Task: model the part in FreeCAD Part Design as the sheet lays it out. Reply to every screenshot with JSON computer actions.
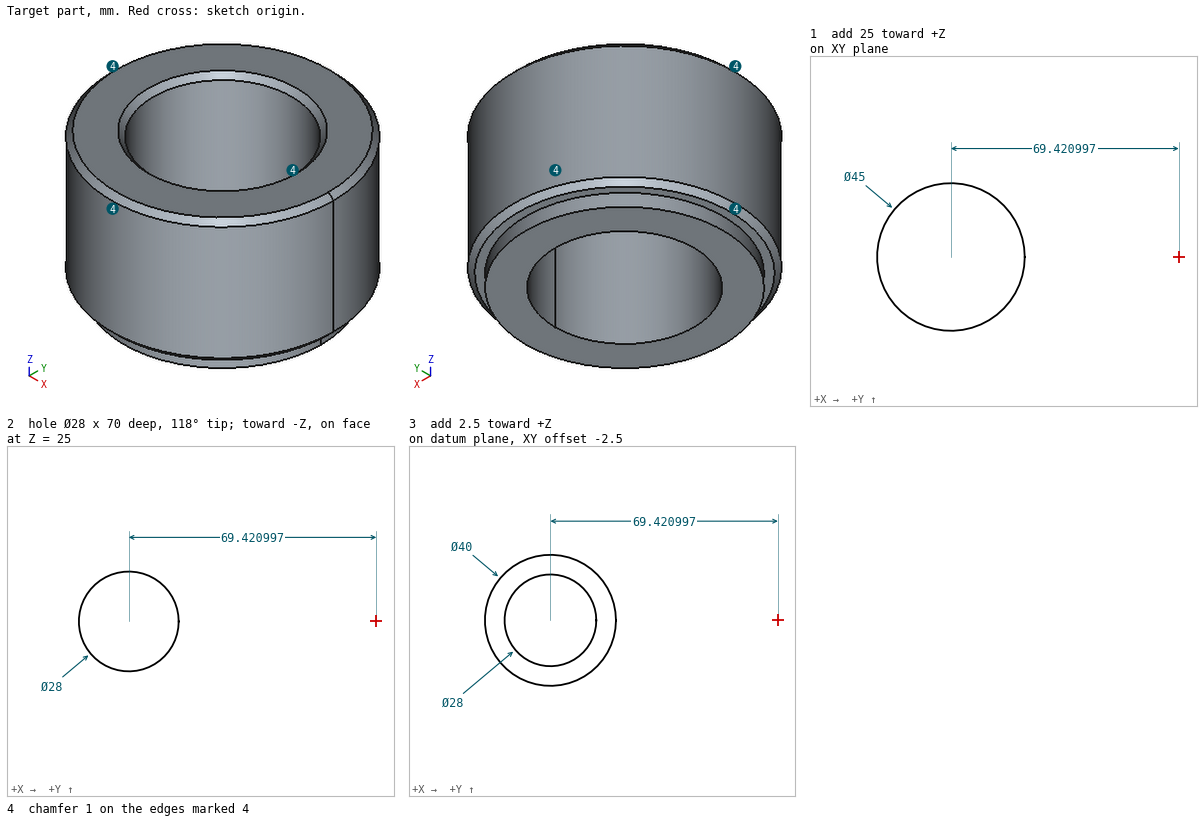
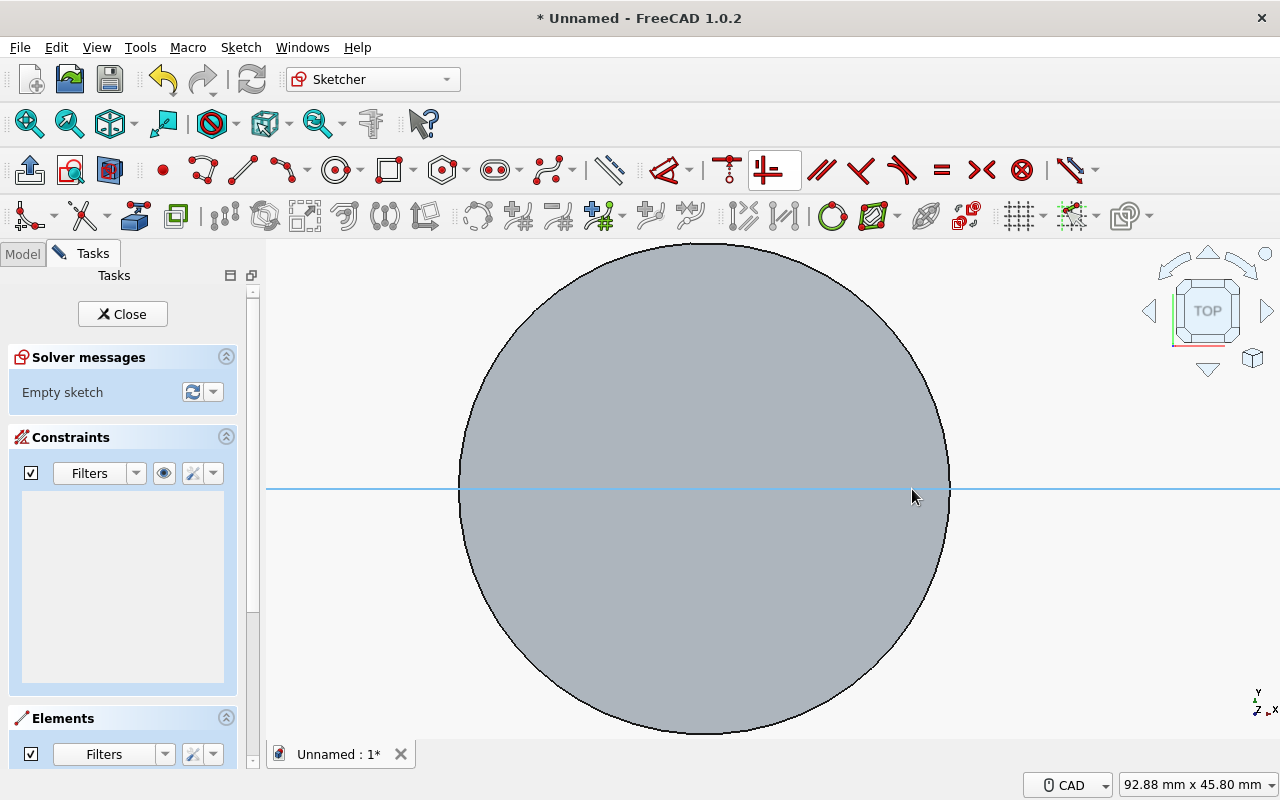
{"action": "key", "text": "g c"}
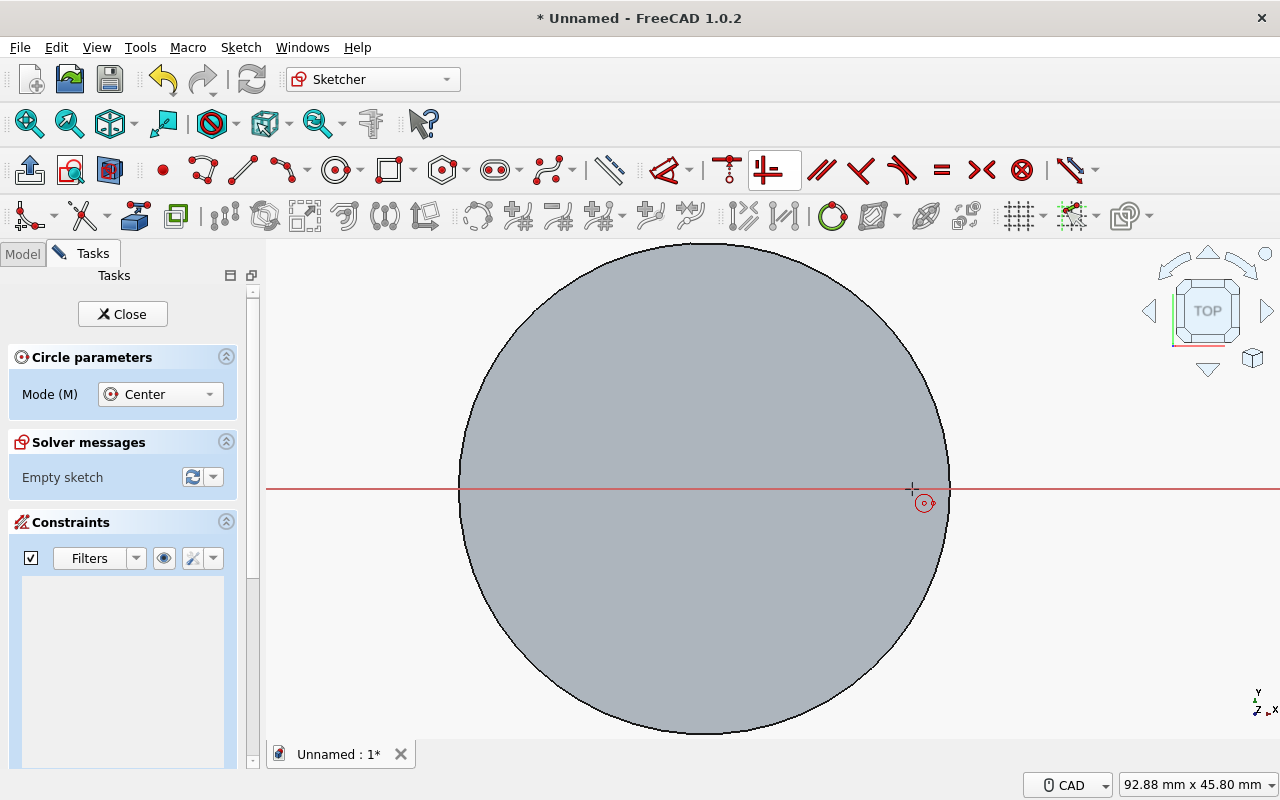
{"action": "left_click", "coordinate": [704, 489]}
{"action": "mouse_move", "coordinate": [812, 381]}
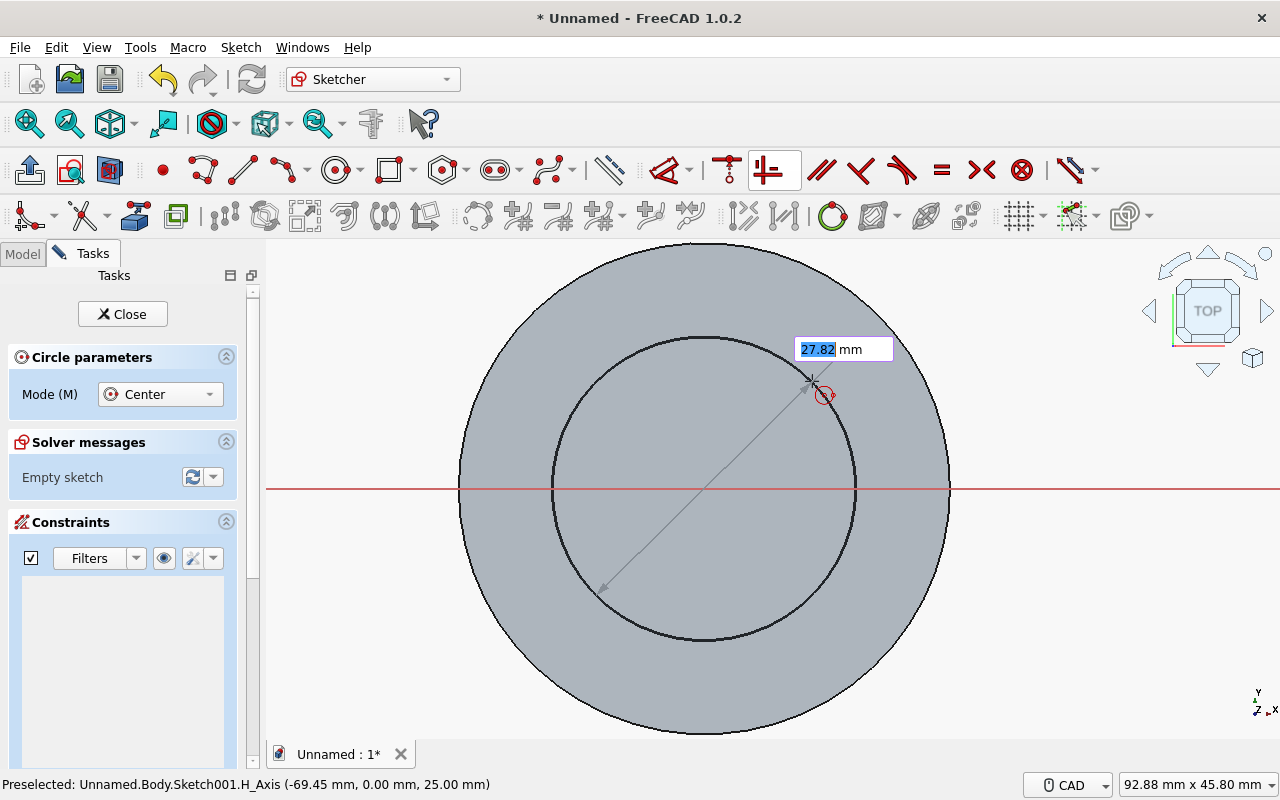
{"action": "type", "text": "28"}
{"action": "key", "text": "Return"}
{"action": "key", "text": "Escape"}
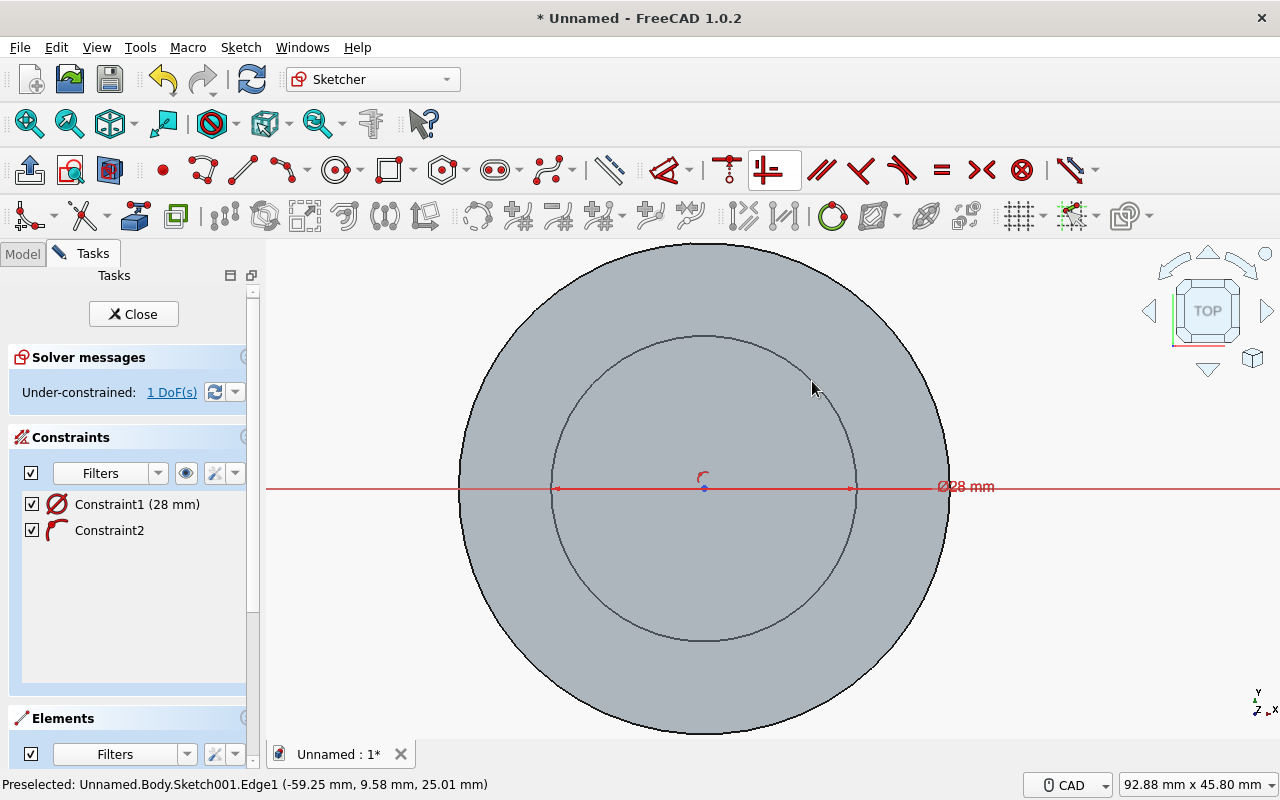
{"action": "key", "text": "d"}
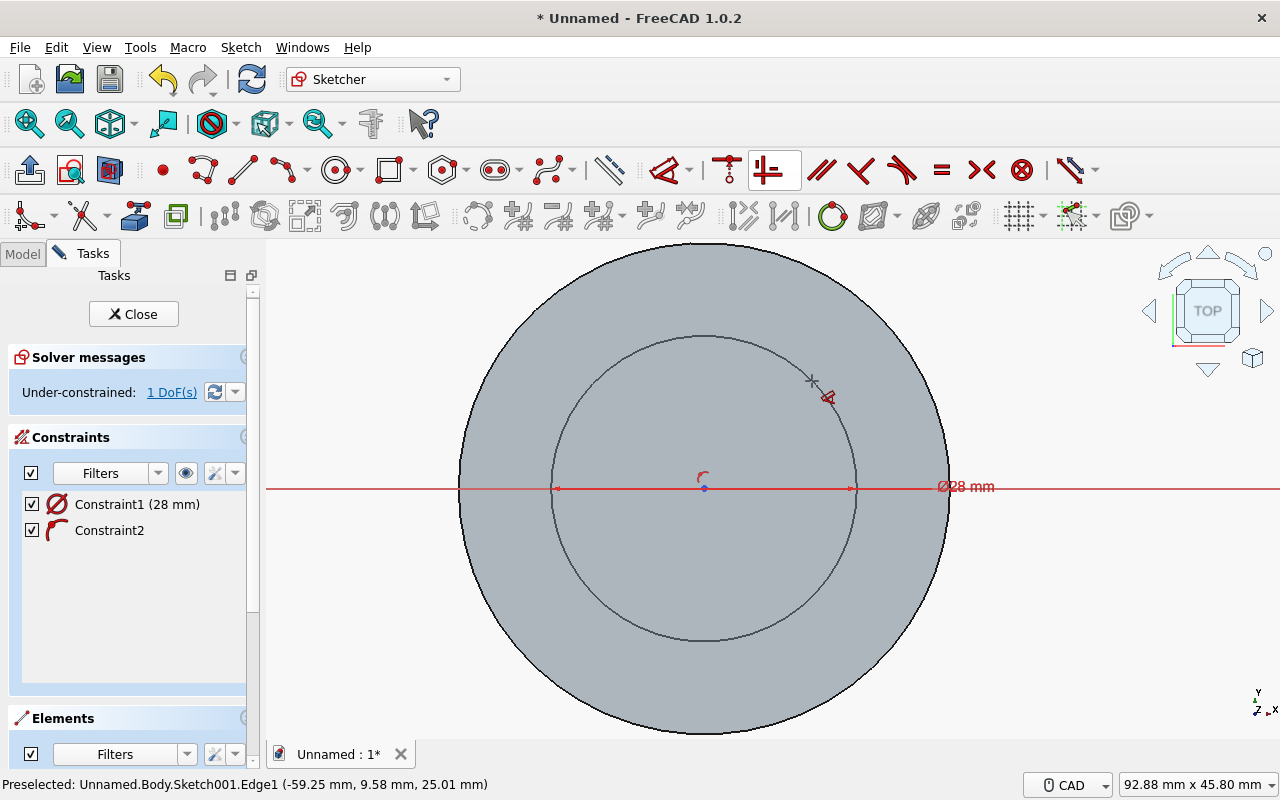
{"action": "left_click", "coordinate": [704, 489]}
{"action": "left_click", "coordinate": [909, 523]}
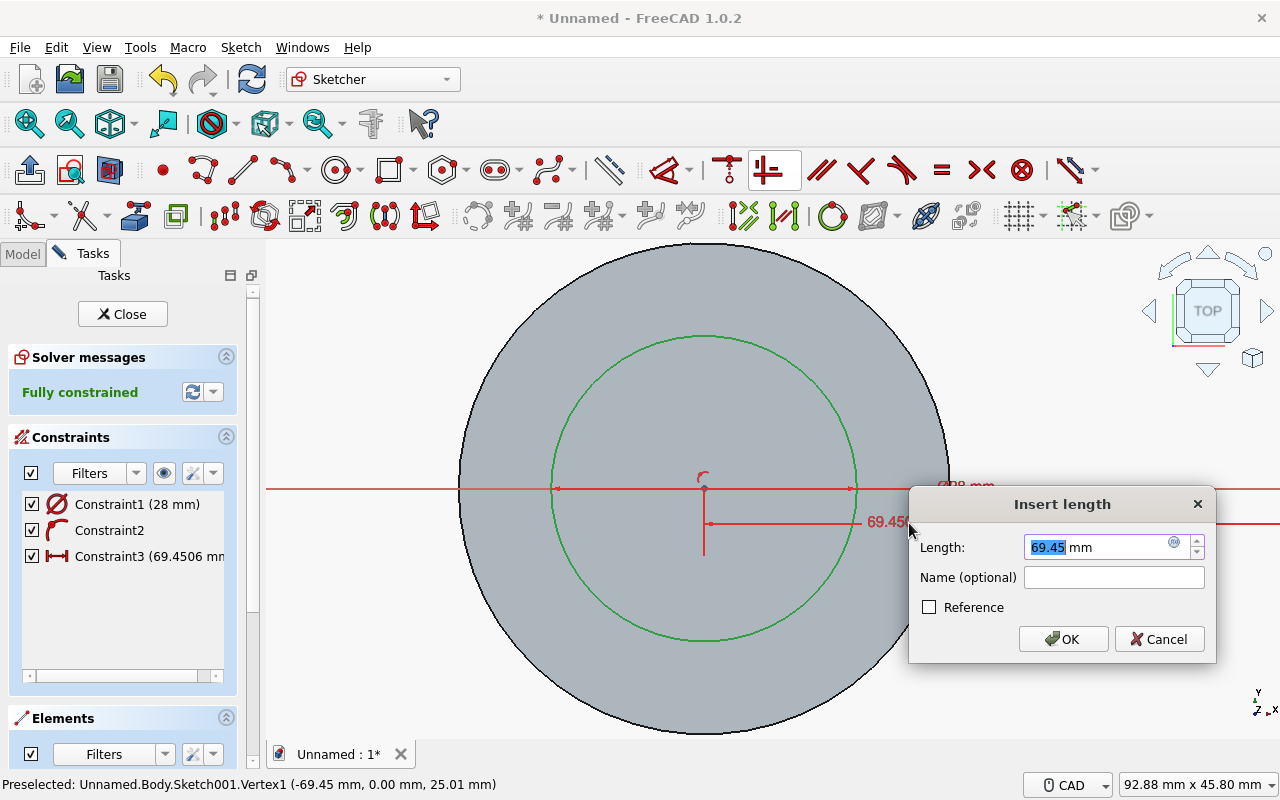
{"action": "type", "text": "69.420997"}
{"action": "key", "text": "Return"}
{"action": "key", "text": "Escape"}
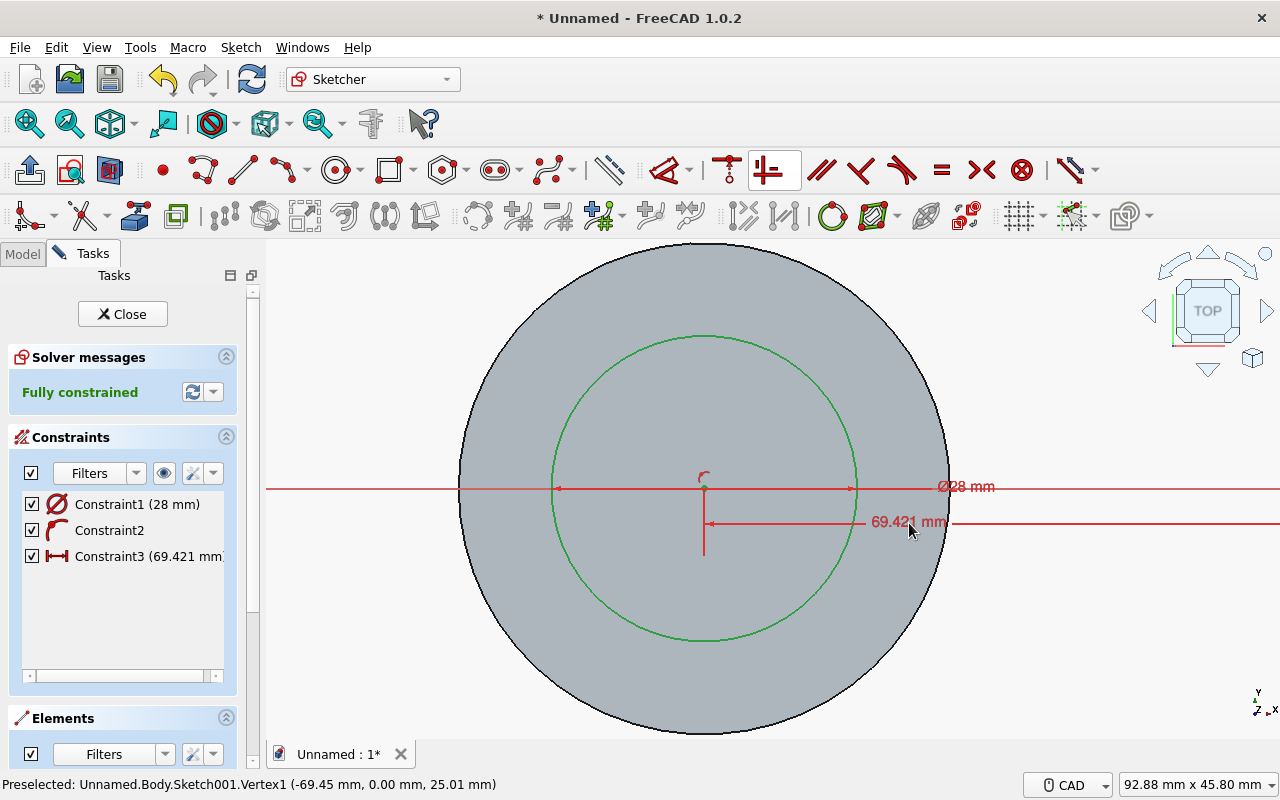
{"action": "left_click", "coordinate": [123, 314]}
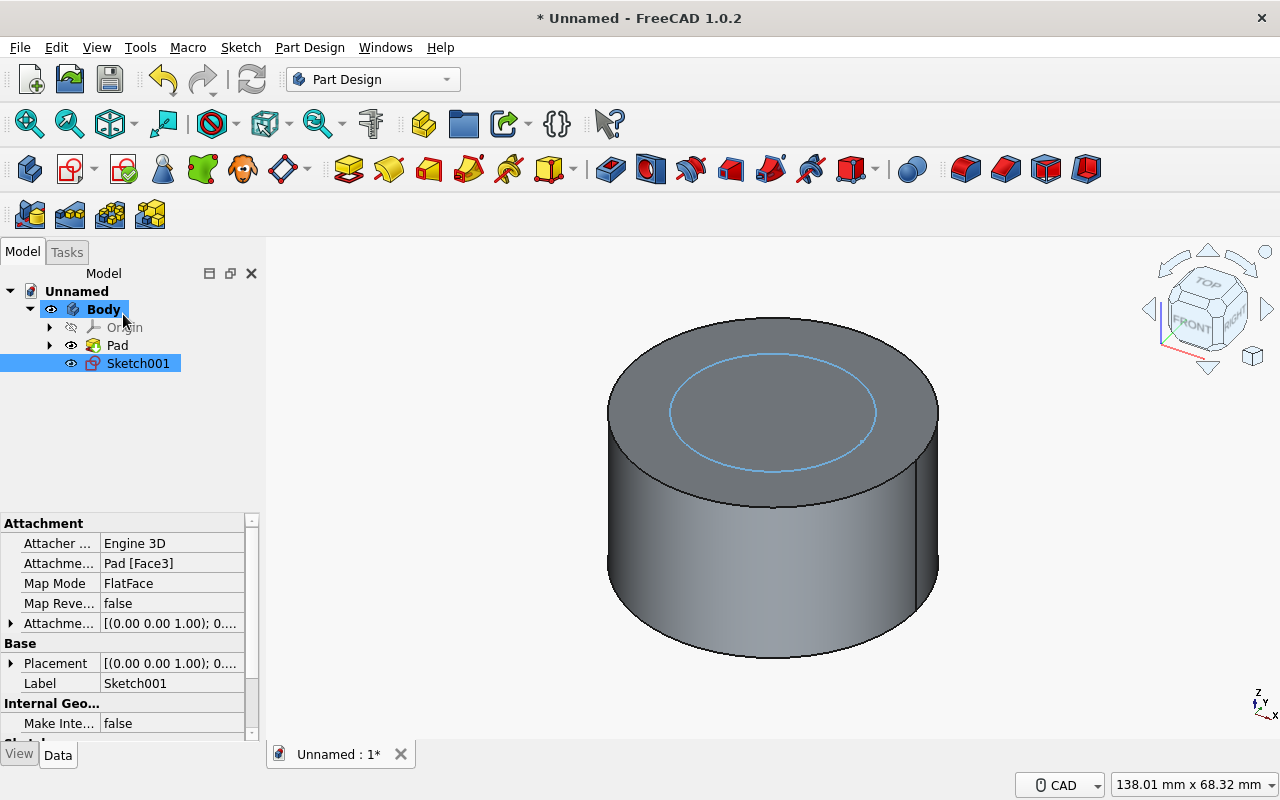
{"action": "left_click", "coordinate": [652, 170]}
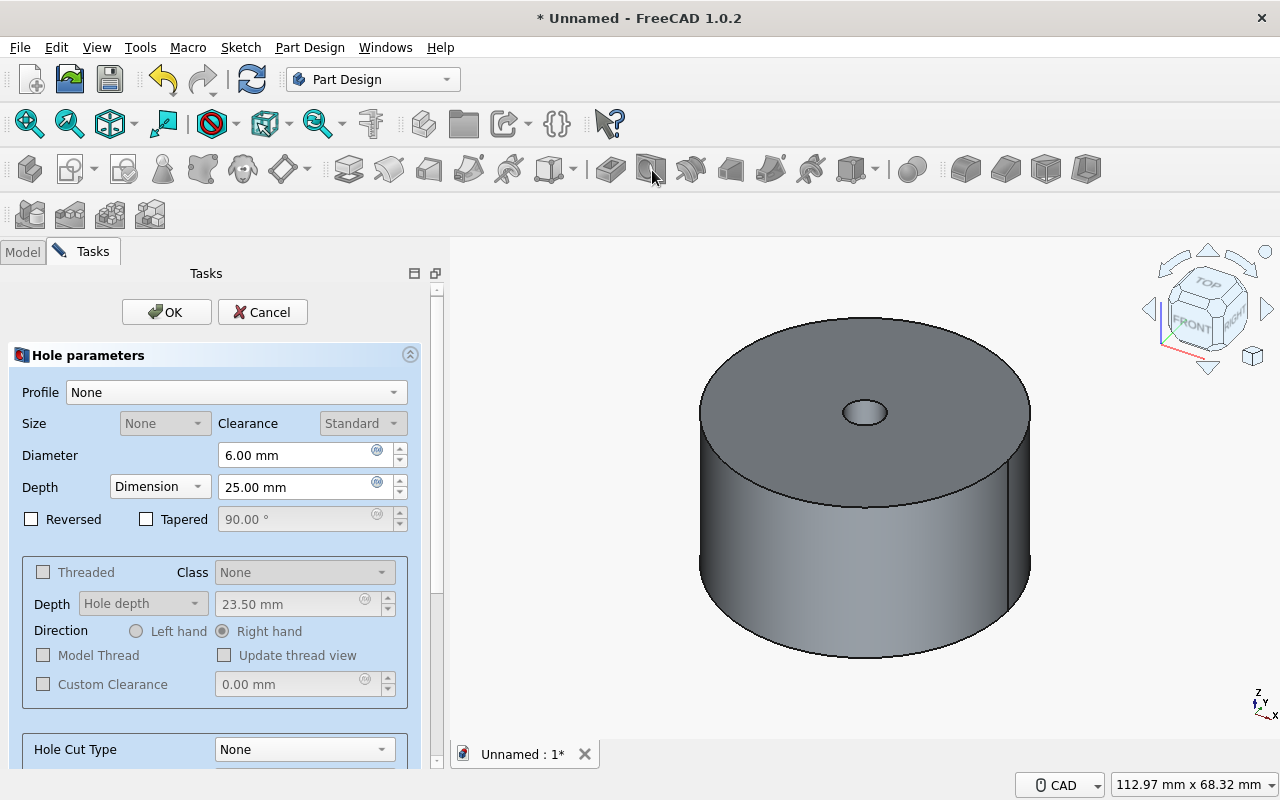
{"action": "triple_click", "coordinate": [305, 455]}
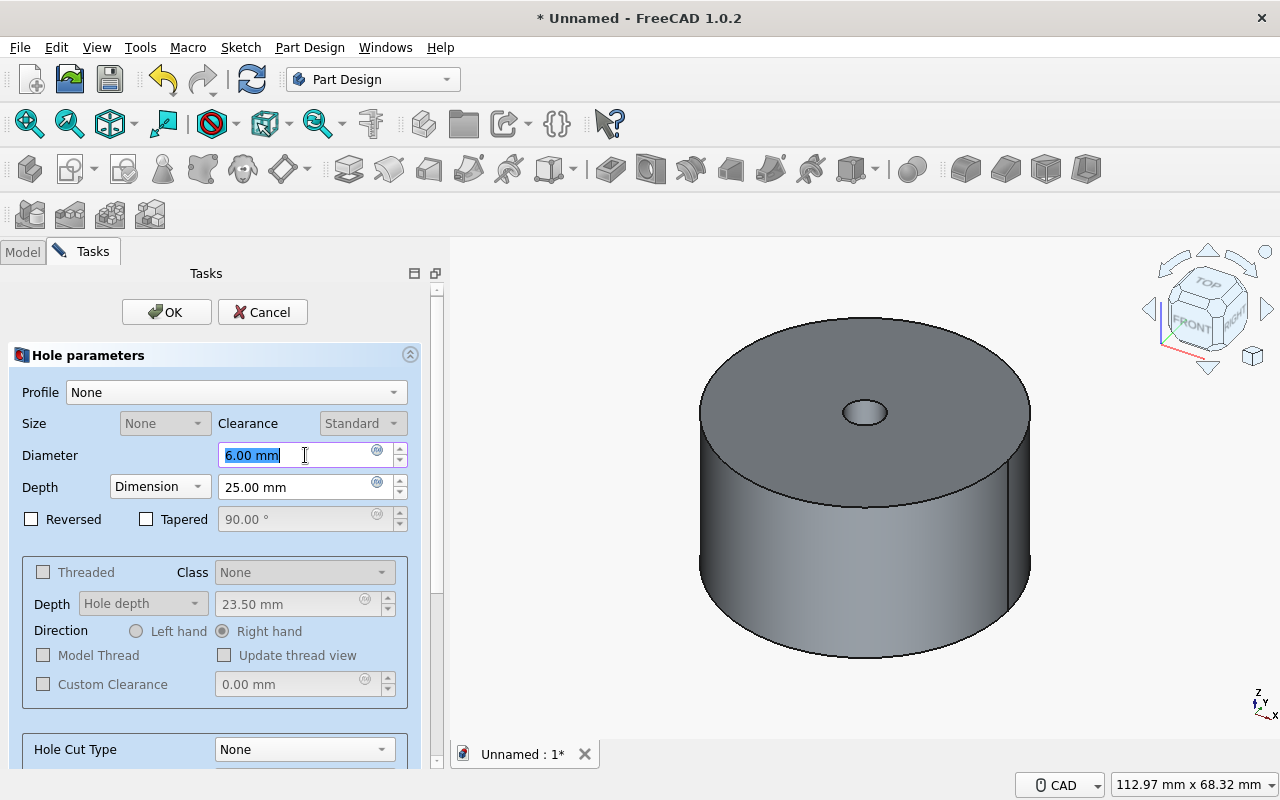
{"action": "type", "text": "28"}
{"action": "key", "text": "Tab"}